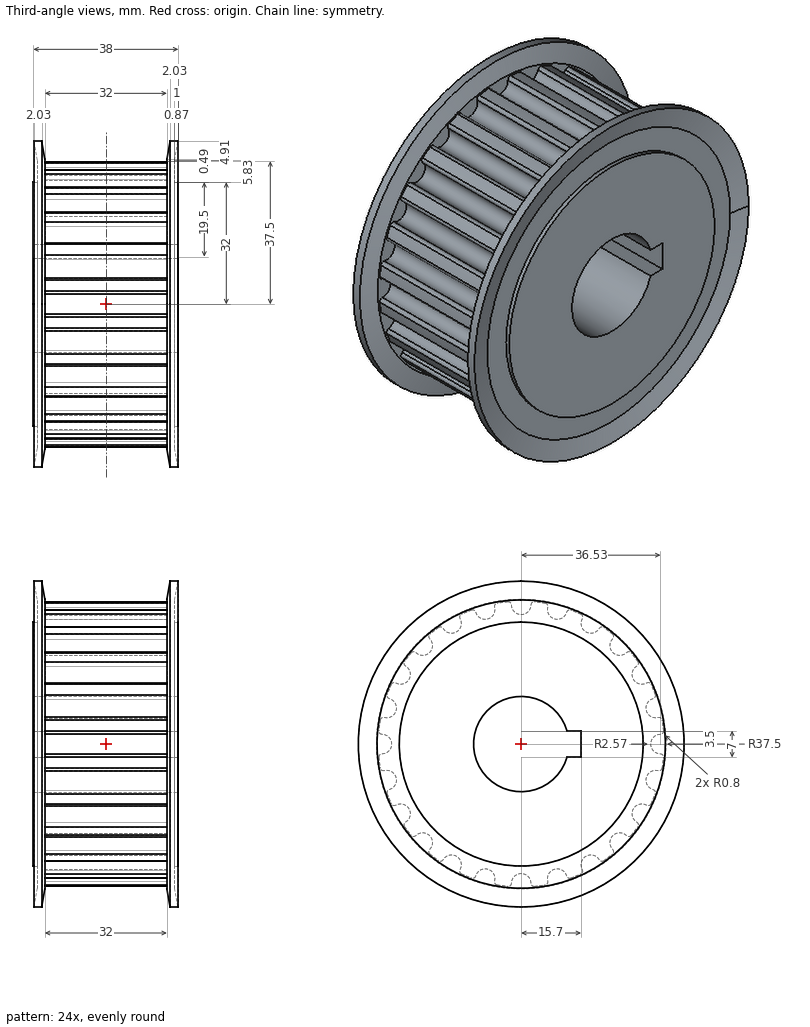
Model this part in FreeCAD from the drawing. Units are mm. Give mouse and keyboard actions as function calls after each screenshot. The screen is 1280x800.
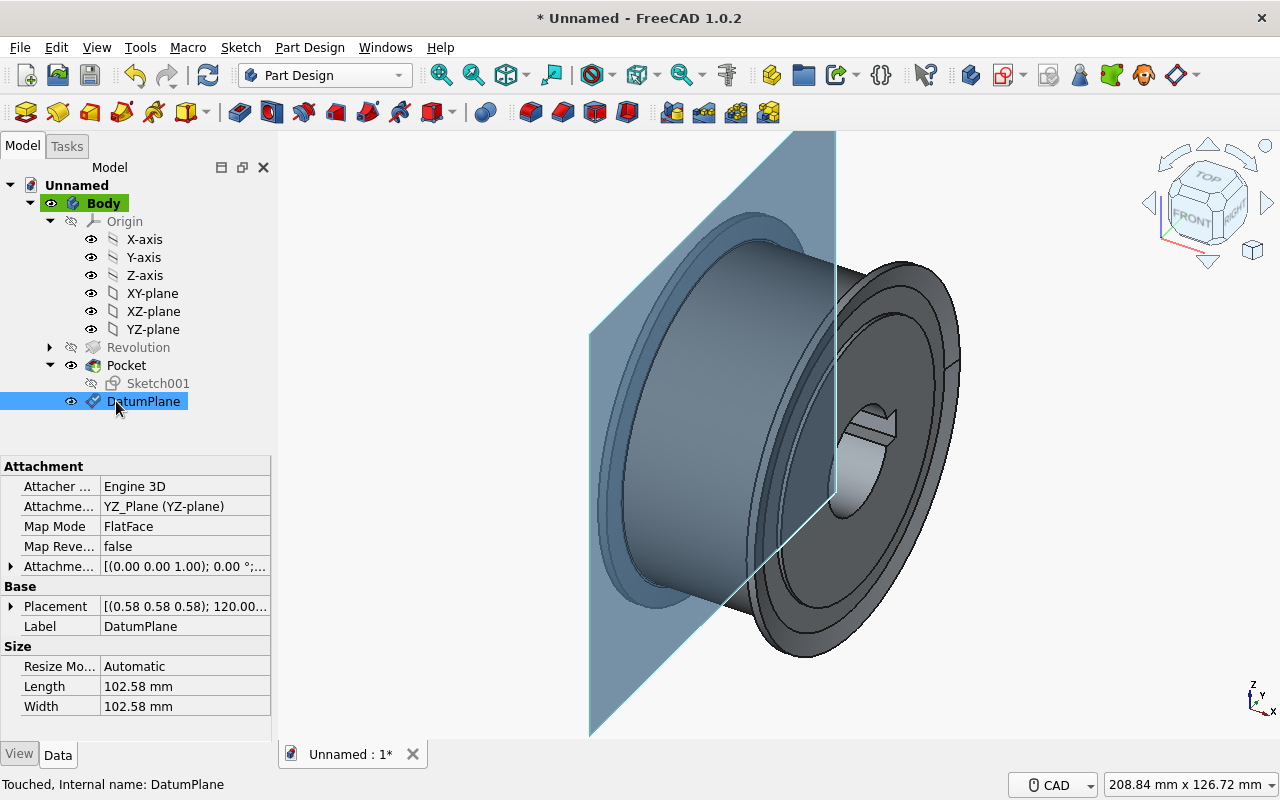
click(1004, 76)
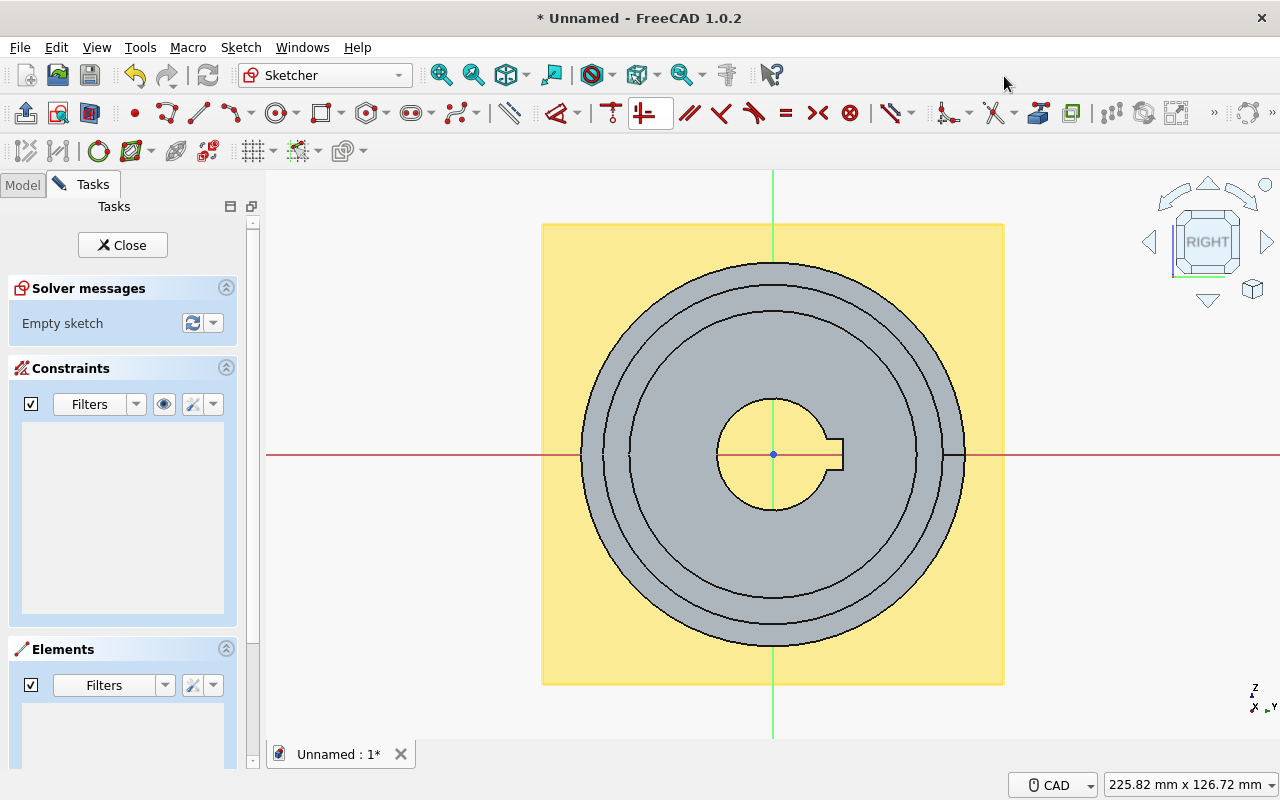
click(90, 114)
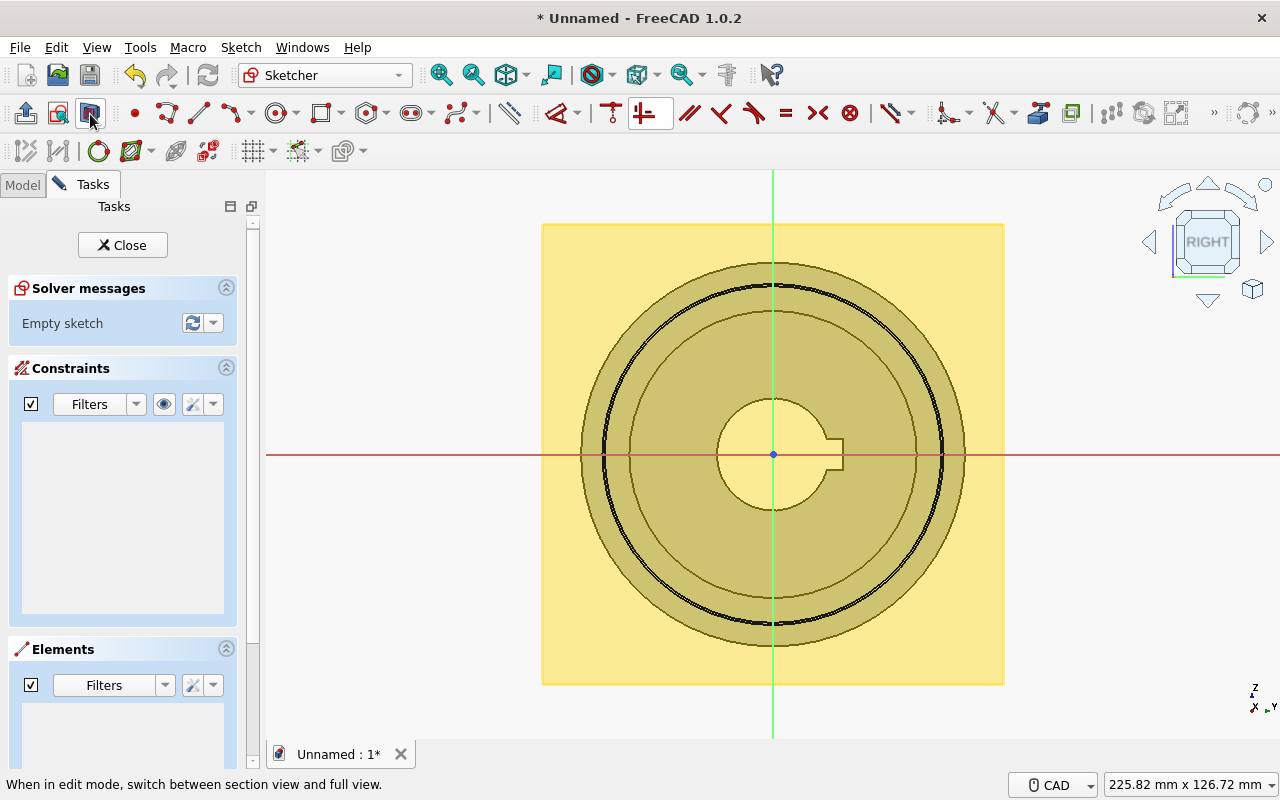
scroll(956, 455, up, 12)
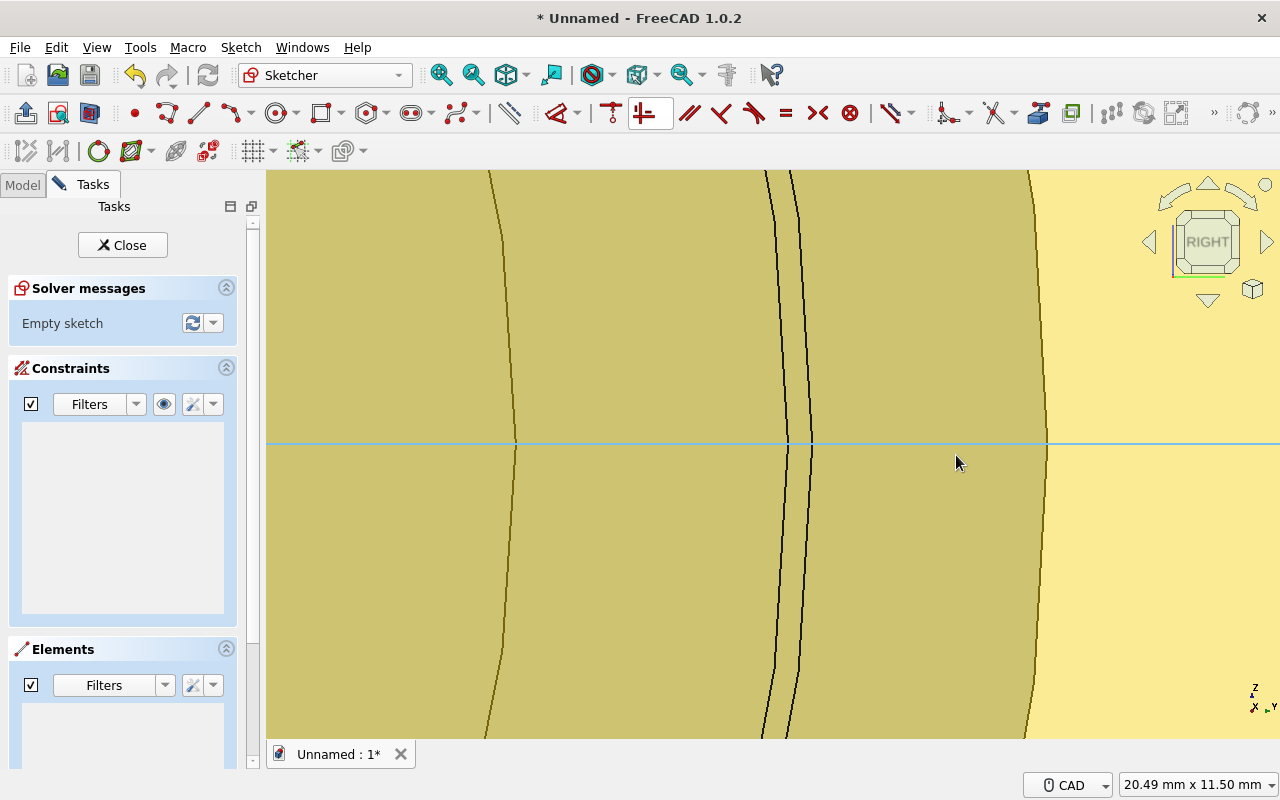
click(232, 114)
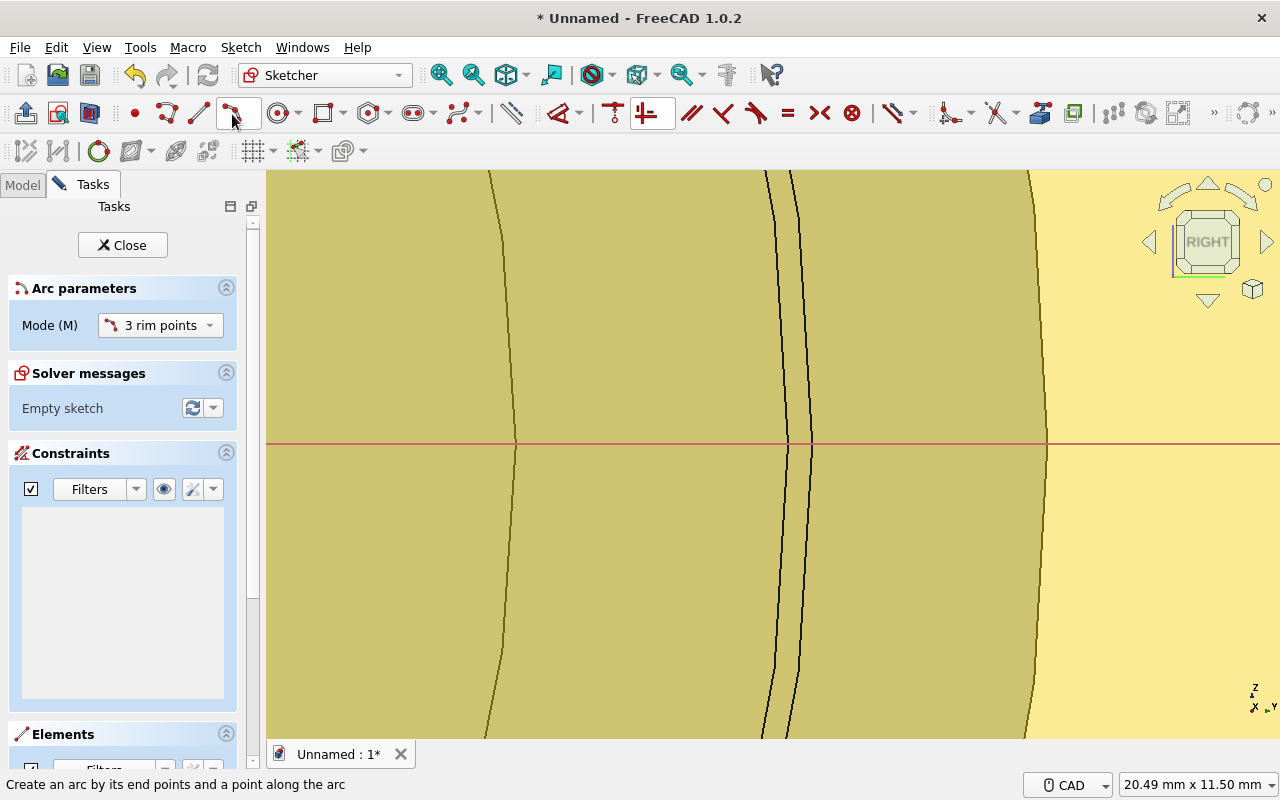
click(741, 317)
click(741, 572)
click(619, 405)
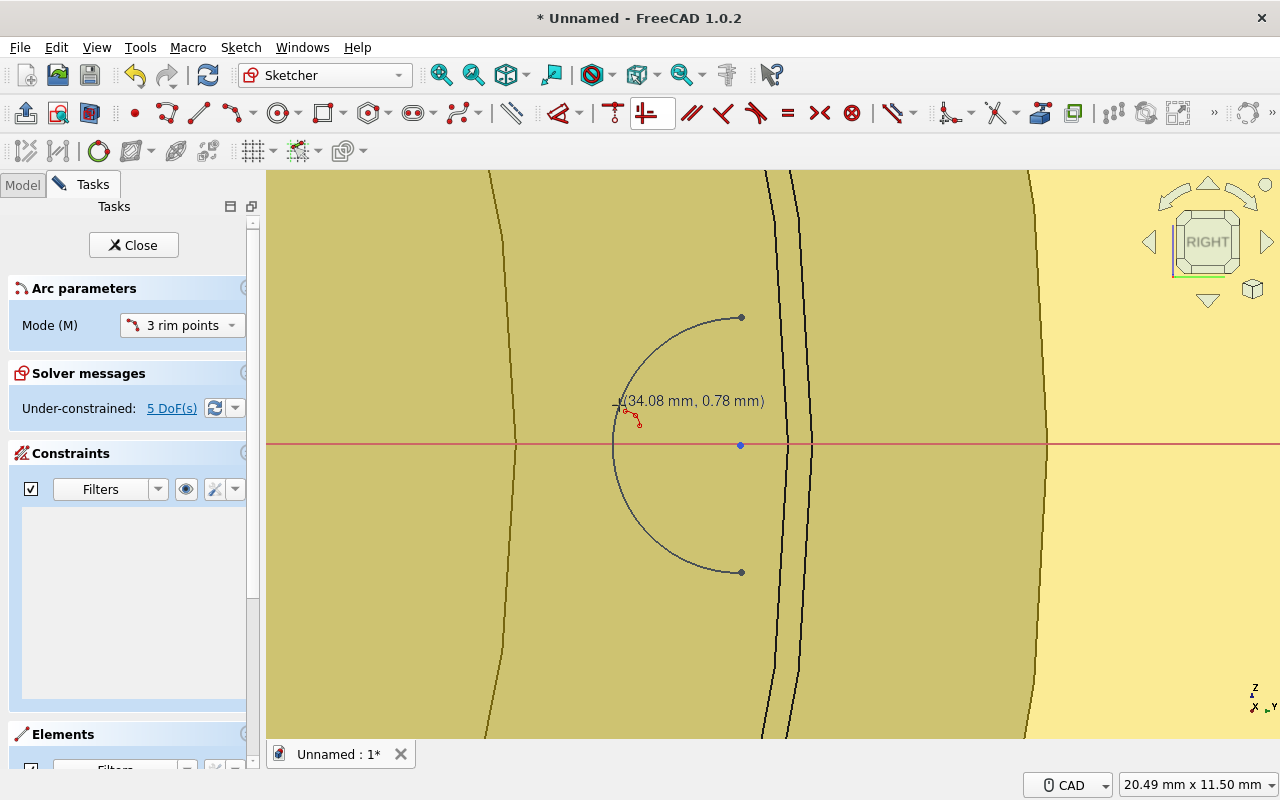
click(741, 573)
click(780, 615)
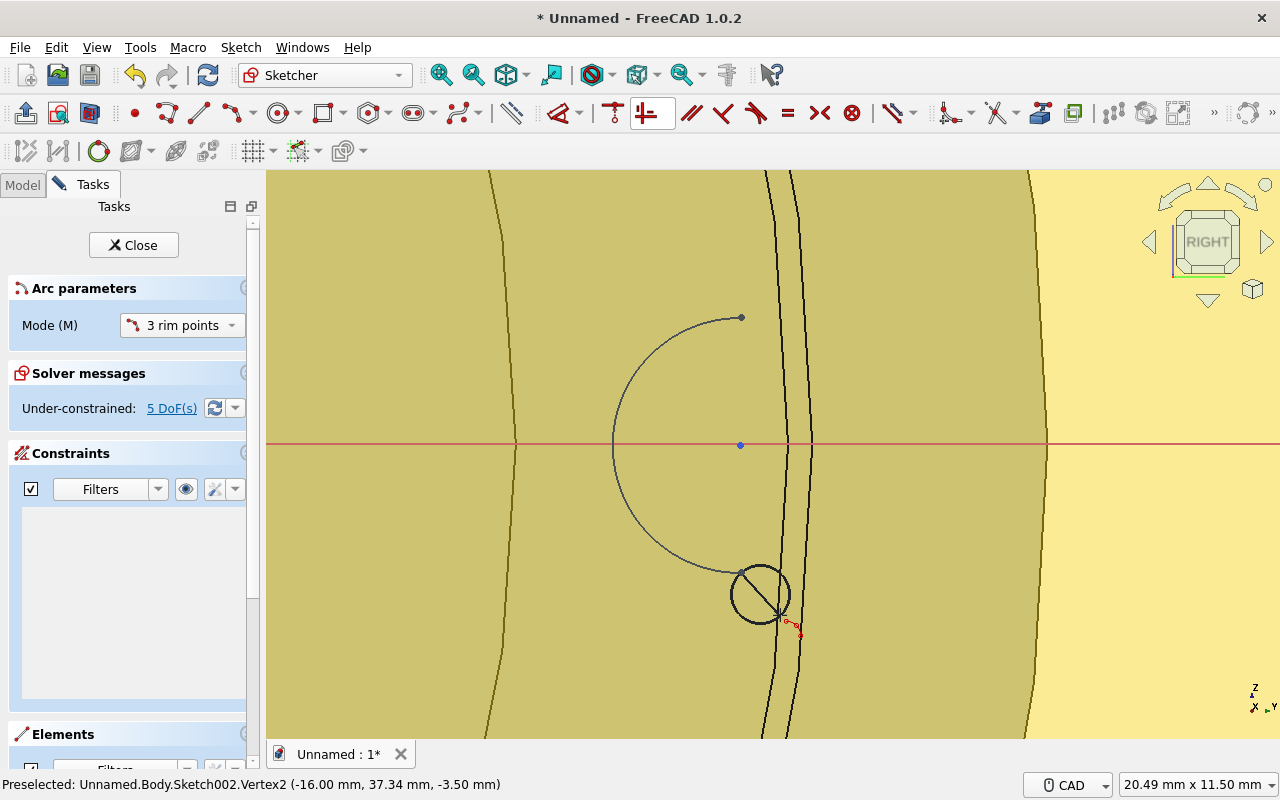
scroll(770, 585, up, 2)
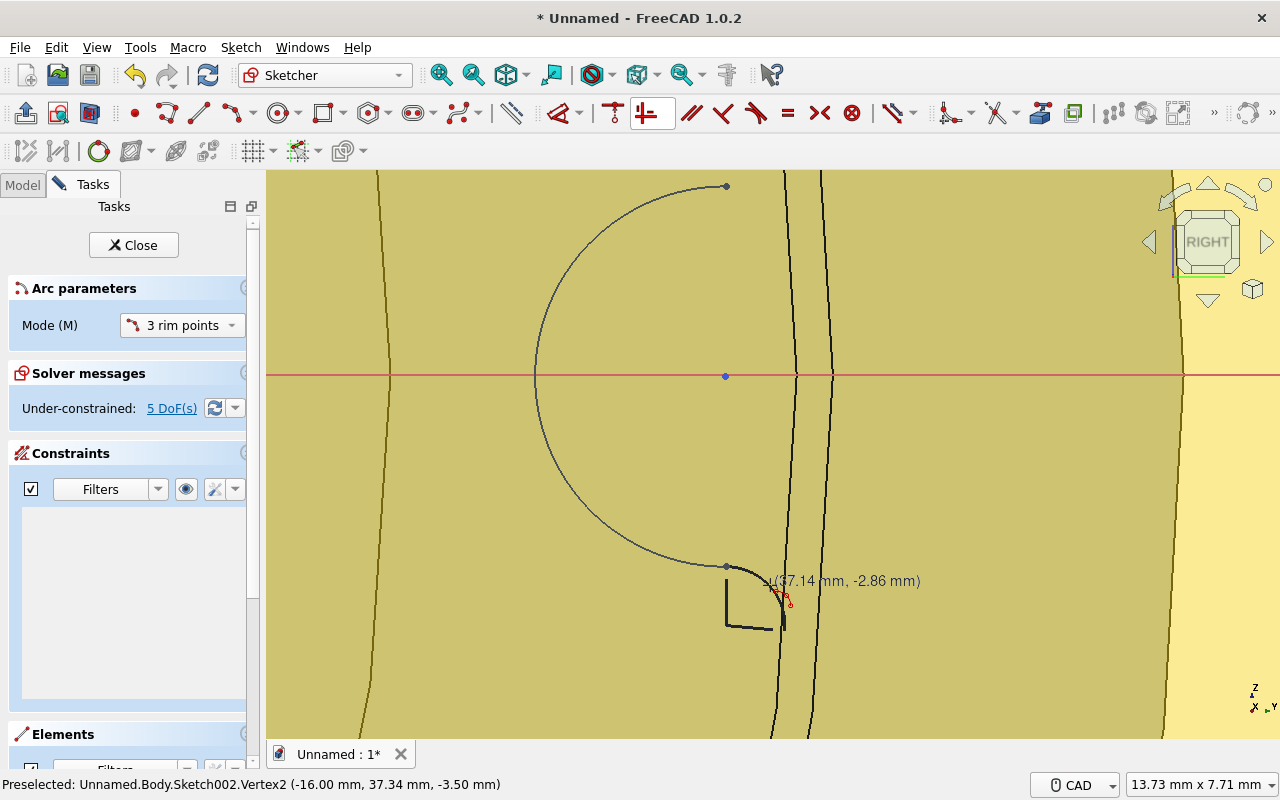
click(770, 584)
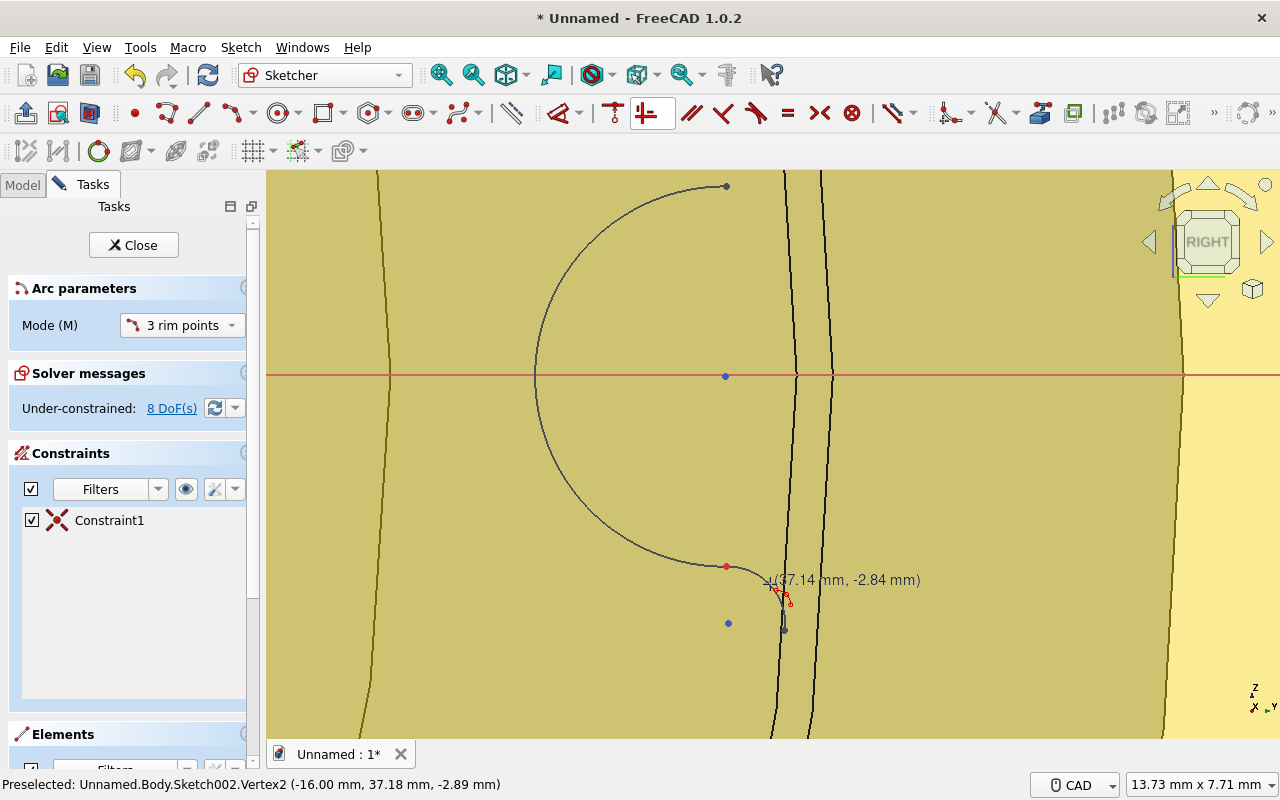
click(785, 631)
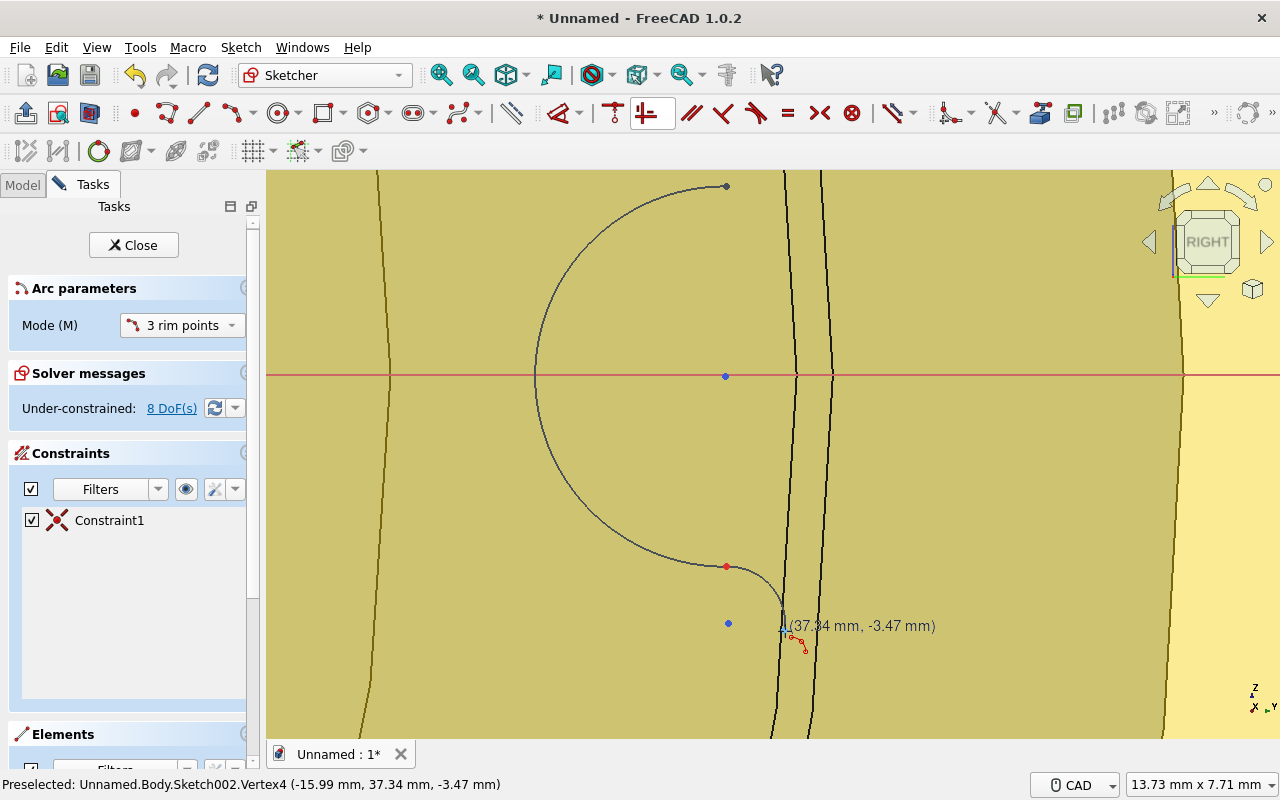
scroll(783, 616, down, 2)